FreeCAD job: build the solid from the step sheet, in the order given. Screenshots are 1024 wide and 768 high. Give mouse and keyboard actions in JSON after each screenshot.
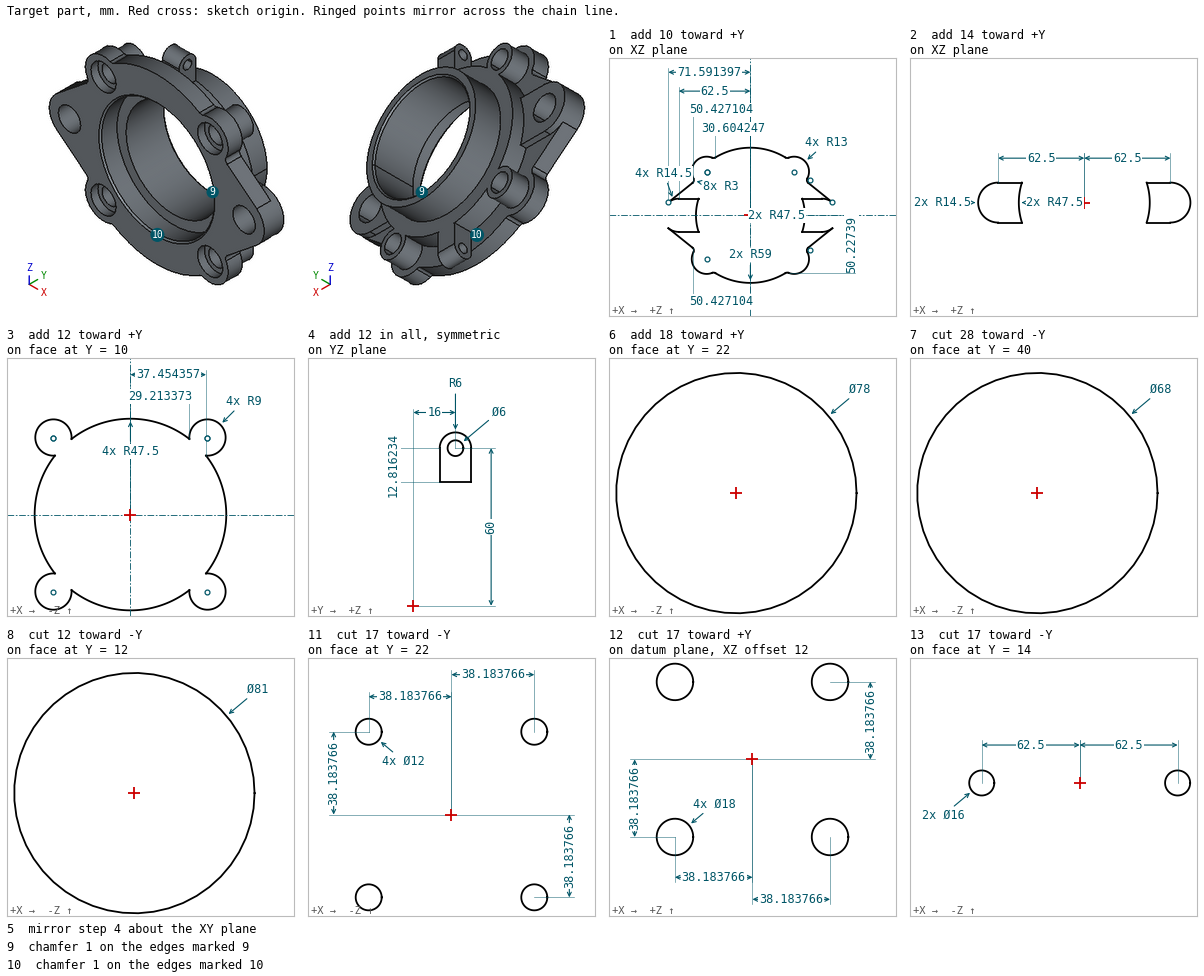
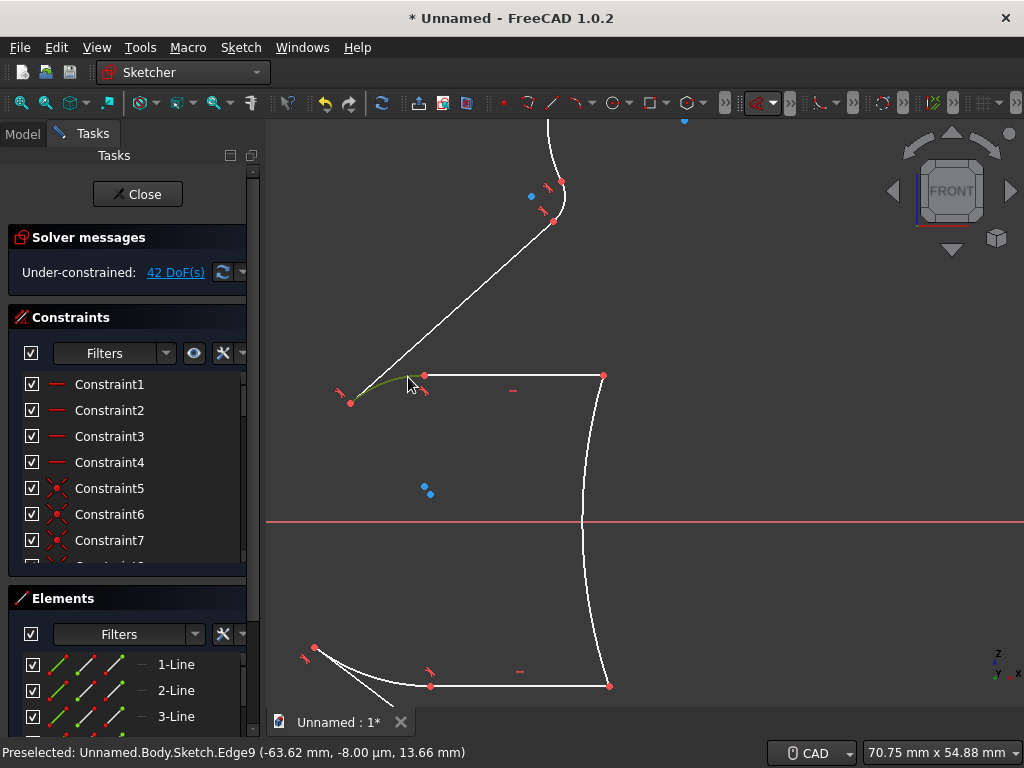
{"action": "scroll", "coordinate": [370, 676], "scroll_direction": "up", "scroll_amount": 2}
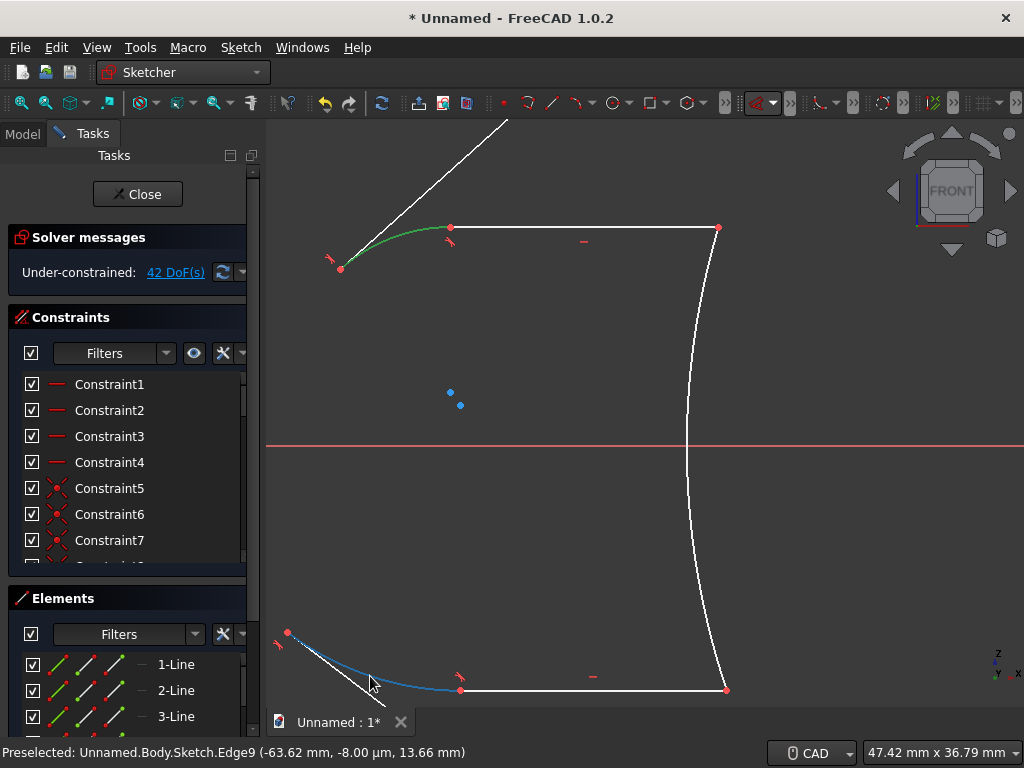
{"action": "left_click", "coordinate": [369, 676]}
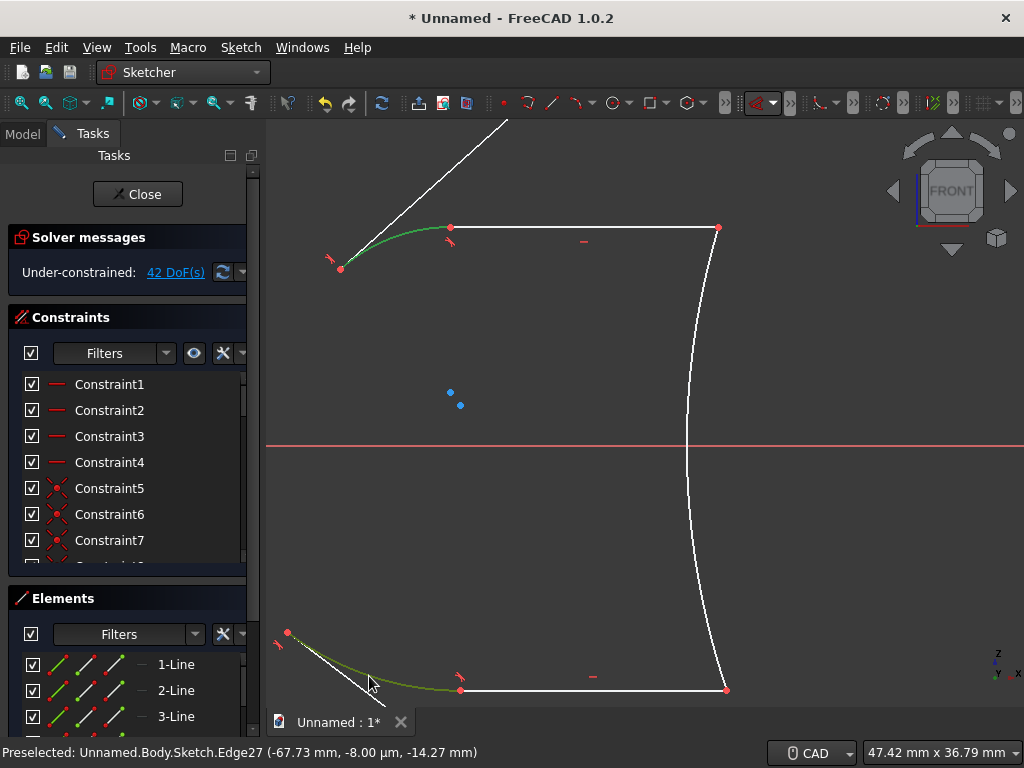
{"action": "key", "text": "c"}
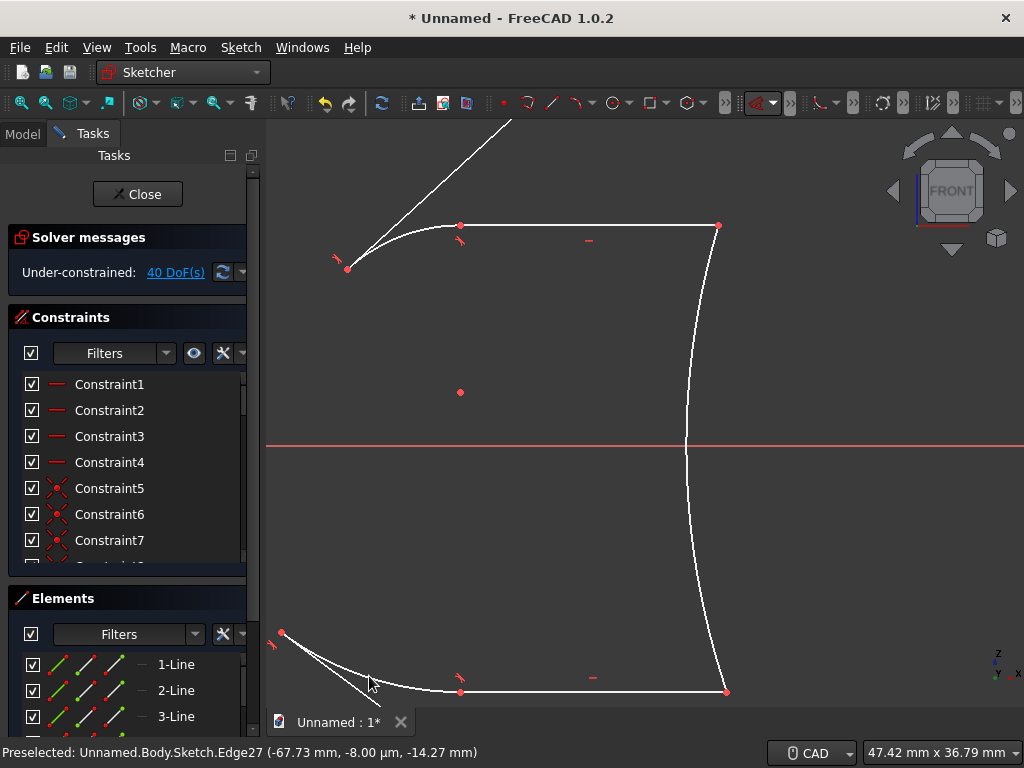
{"action": "scroll", "coordinate": [404, 406], "scroll_direction": "down", "scroll_amount": 9}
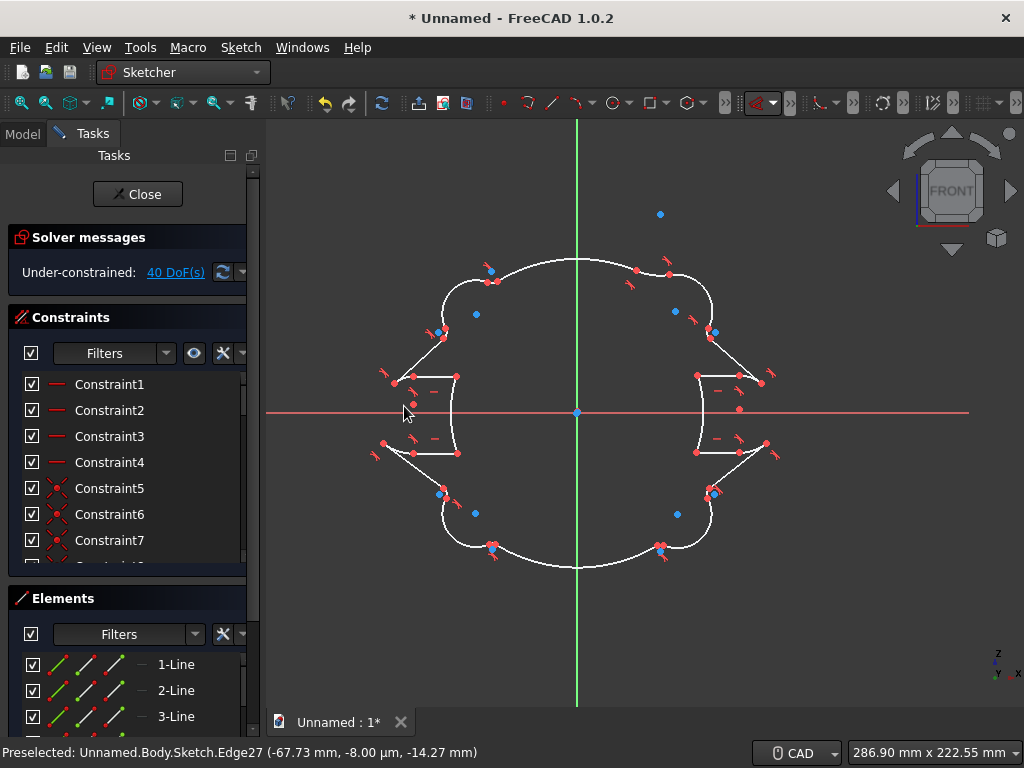
{"action": "left_click", "coordinate": [595, 260]}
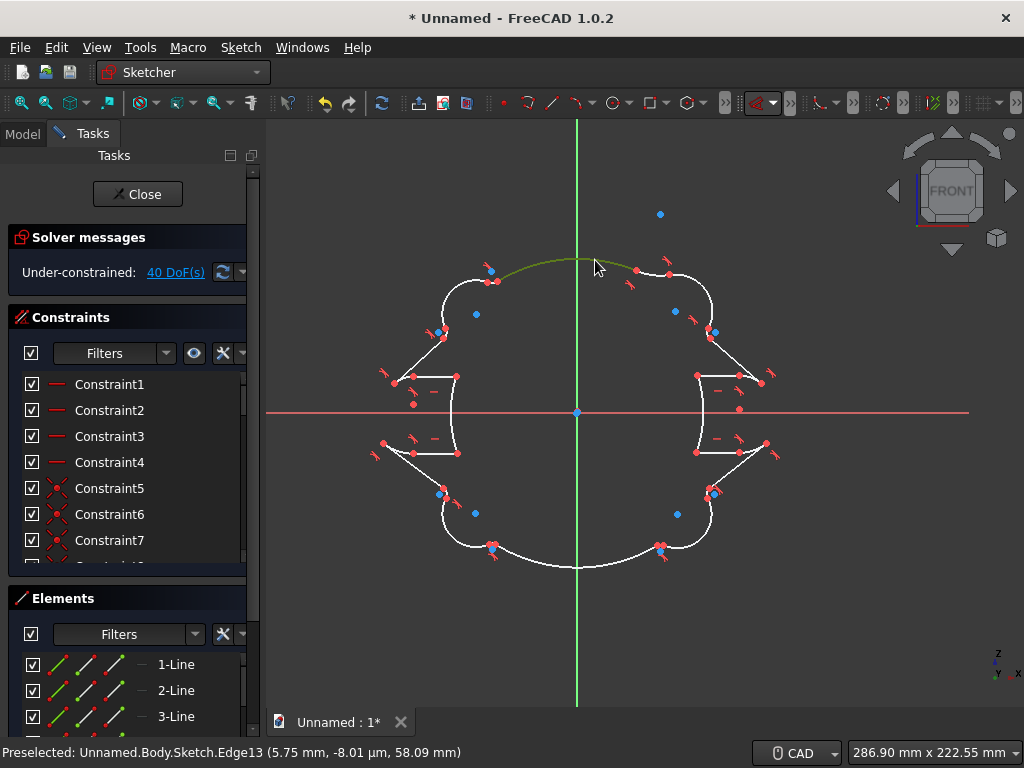
{"action": "left_click", "coordinate": [452, 400]}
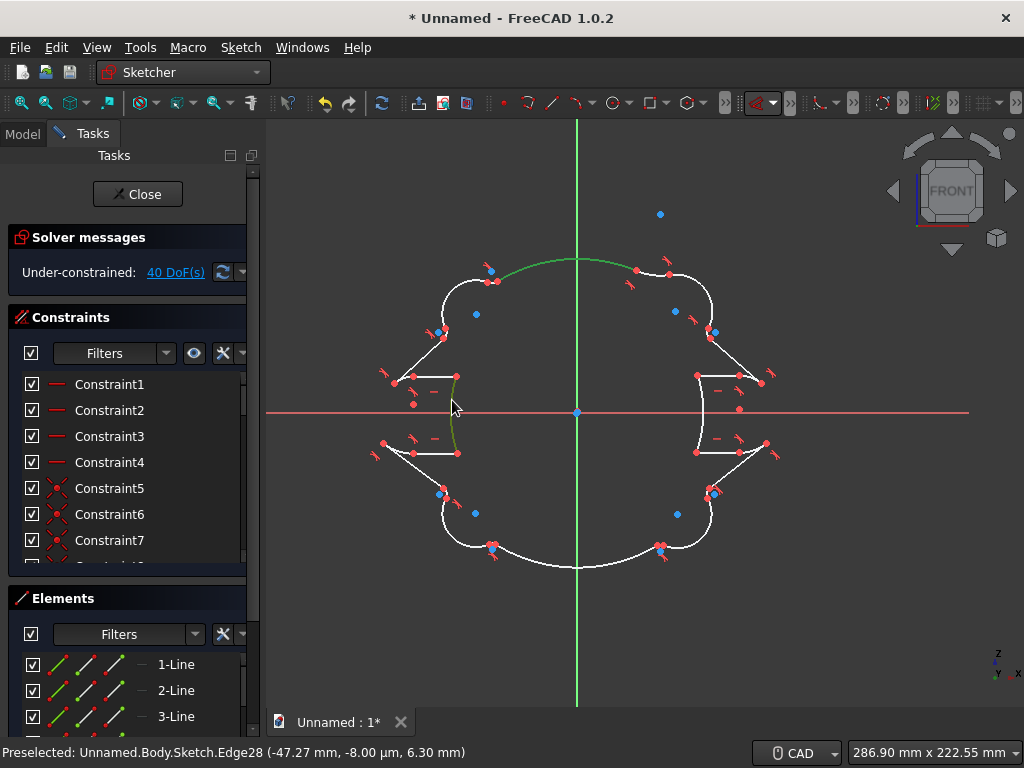
{"action": "key", "text": "c"}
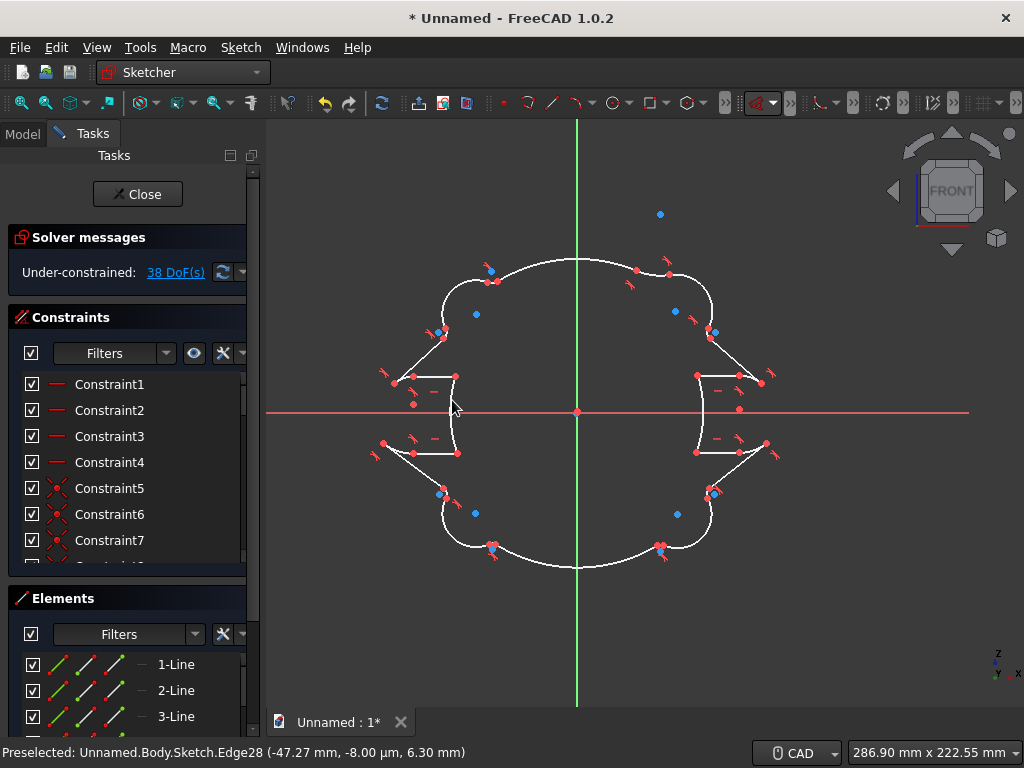
{"action": "scroll", "coordinate": [577, 412], "scroll_direction": "up", "scroll_amount": 10}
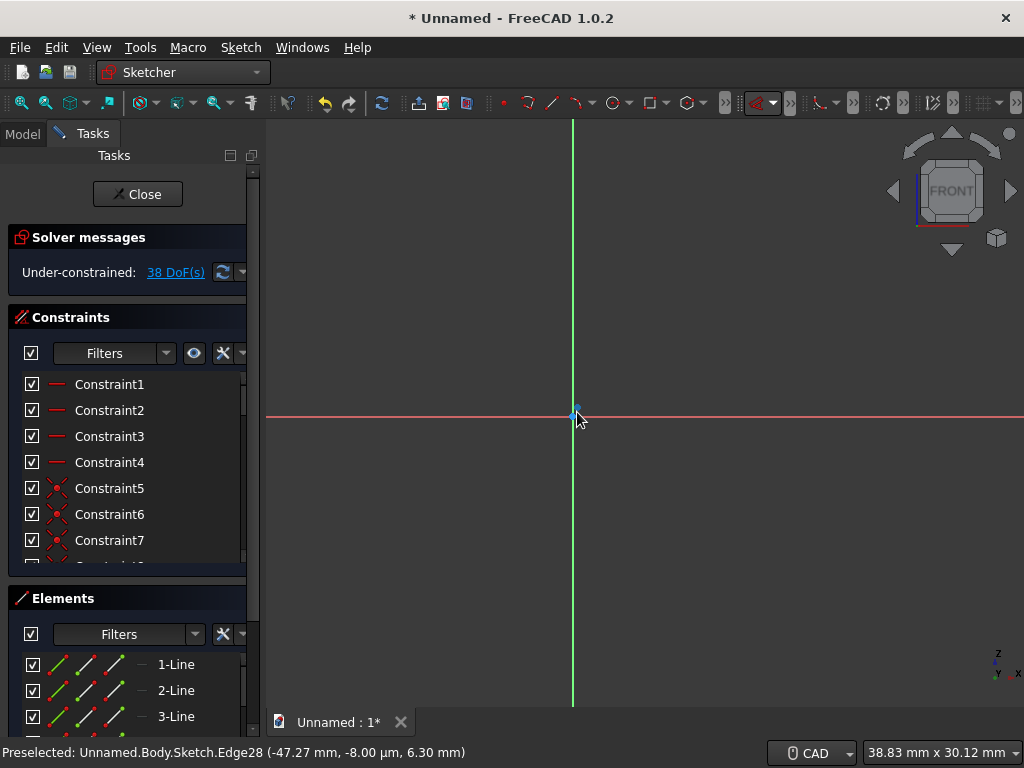
{"action": "left_click_drag", "start_coordinate": [563, 397], "coordinate": [588, 427]}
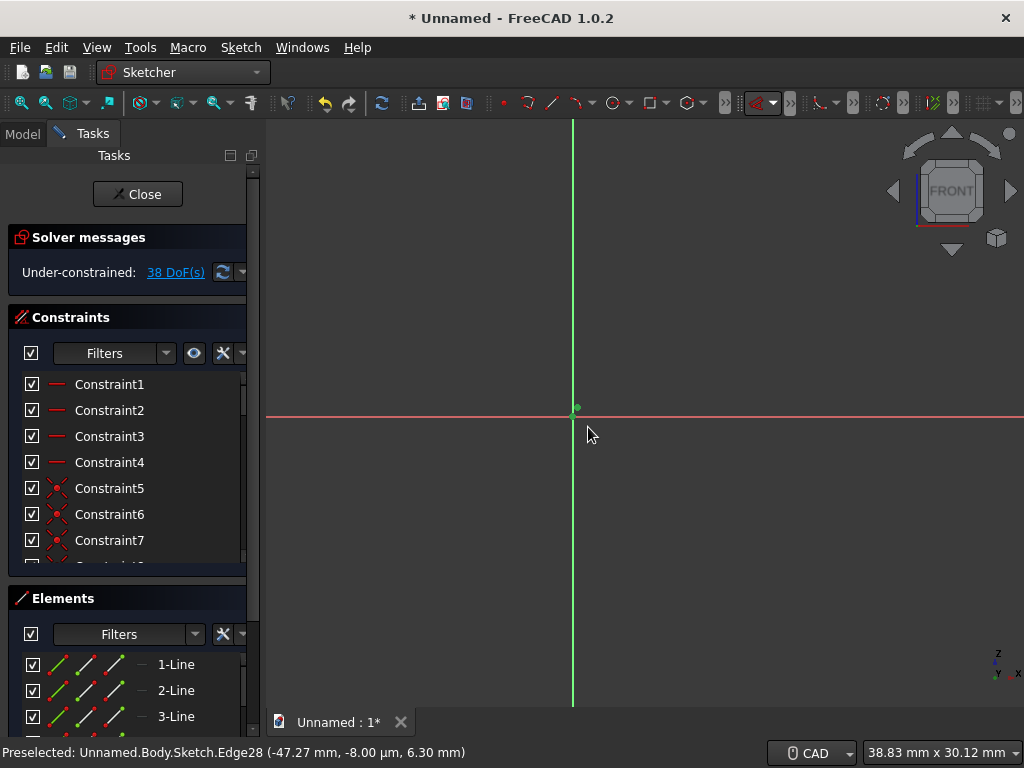
{"action": "key", "text": "c"}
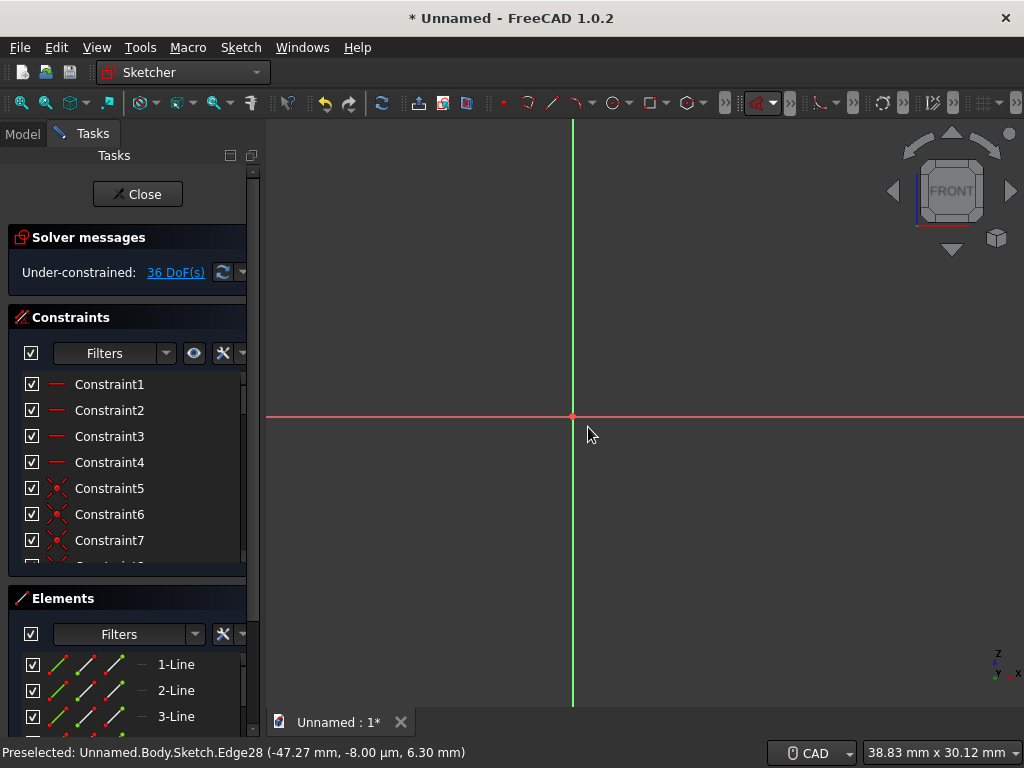
{"action": "scroll", "coordinate": [577, 412], "scroll_direction": "down", "scroll_amount": 10}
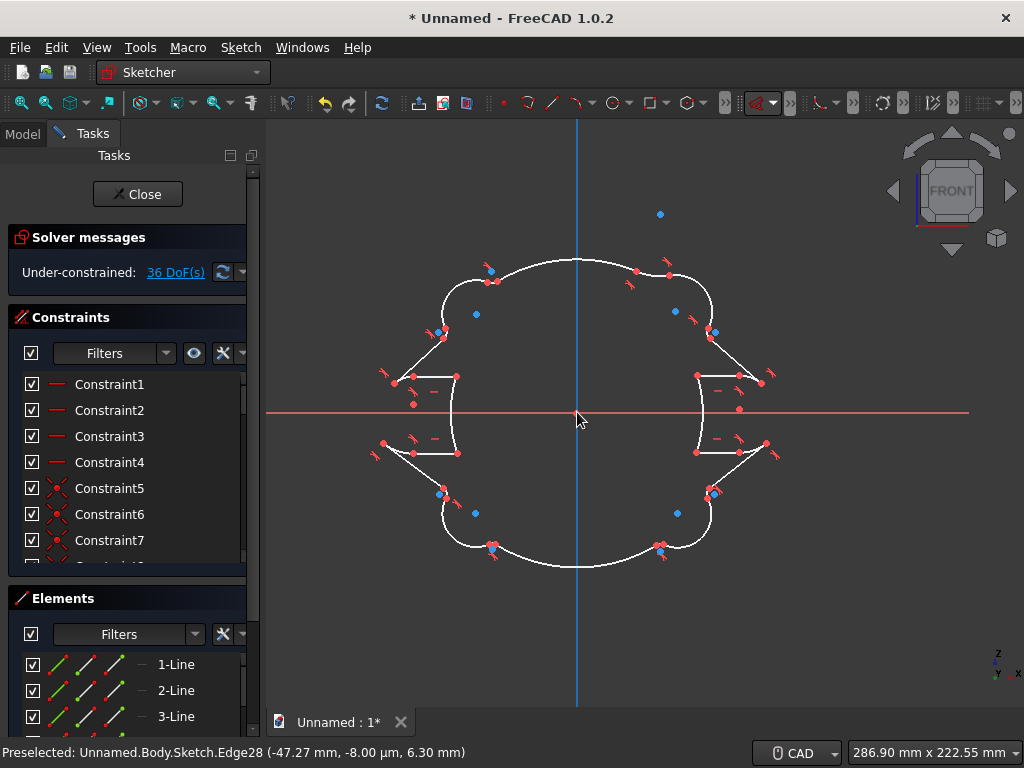
{"action": "scroll", "coordinate": [446, 336], "scroll_direction": "up", "scroll_amount": 8}